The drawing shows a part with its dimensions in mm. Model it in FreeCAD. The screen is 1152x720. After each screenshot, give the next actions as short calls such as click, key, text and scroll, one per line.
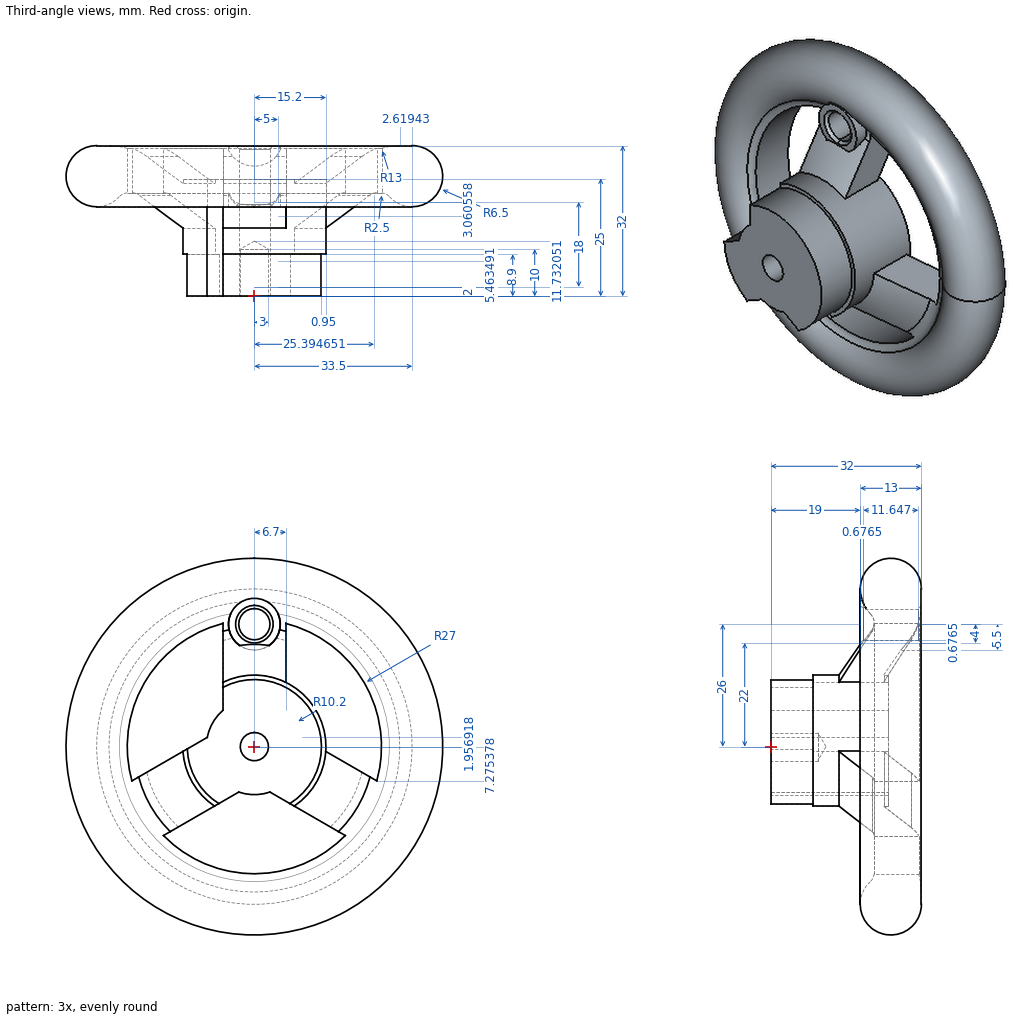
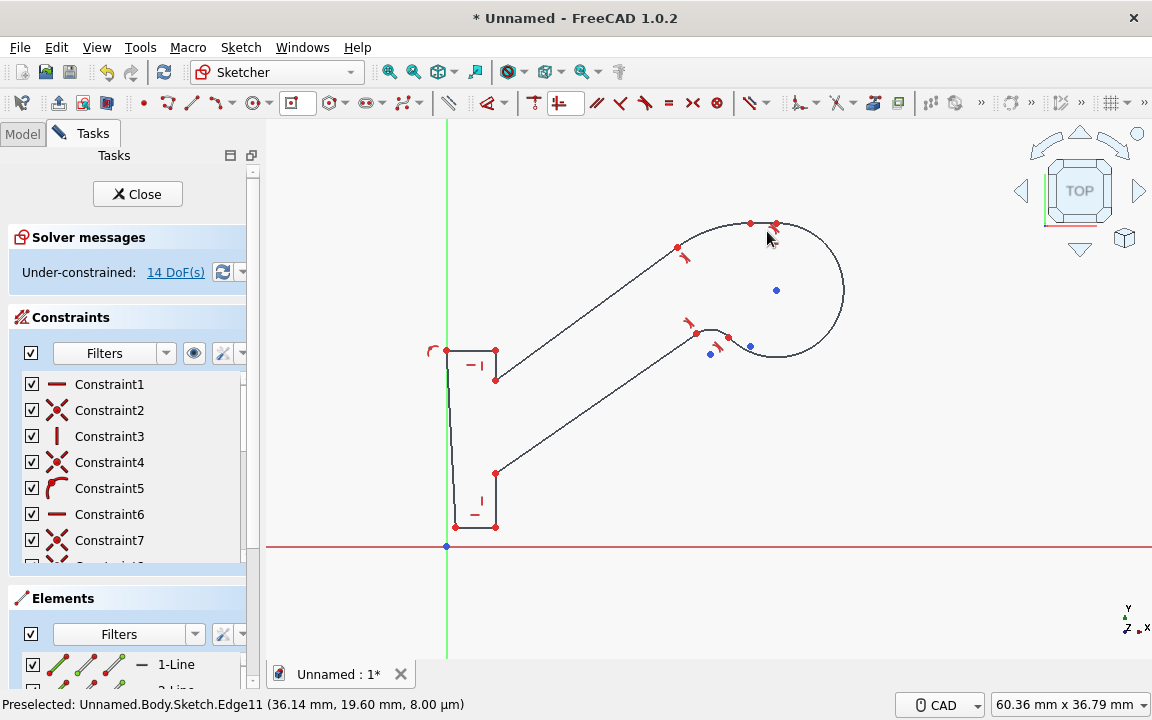
scroll(453, 475, up, 4)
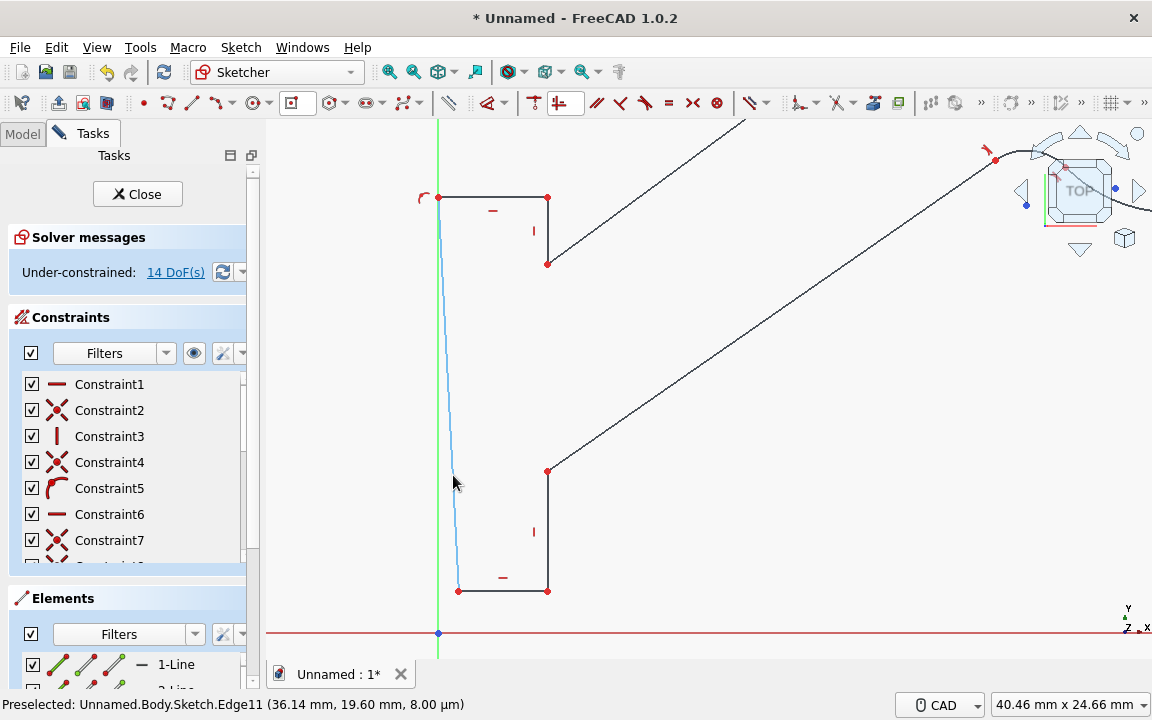
click(453, 473)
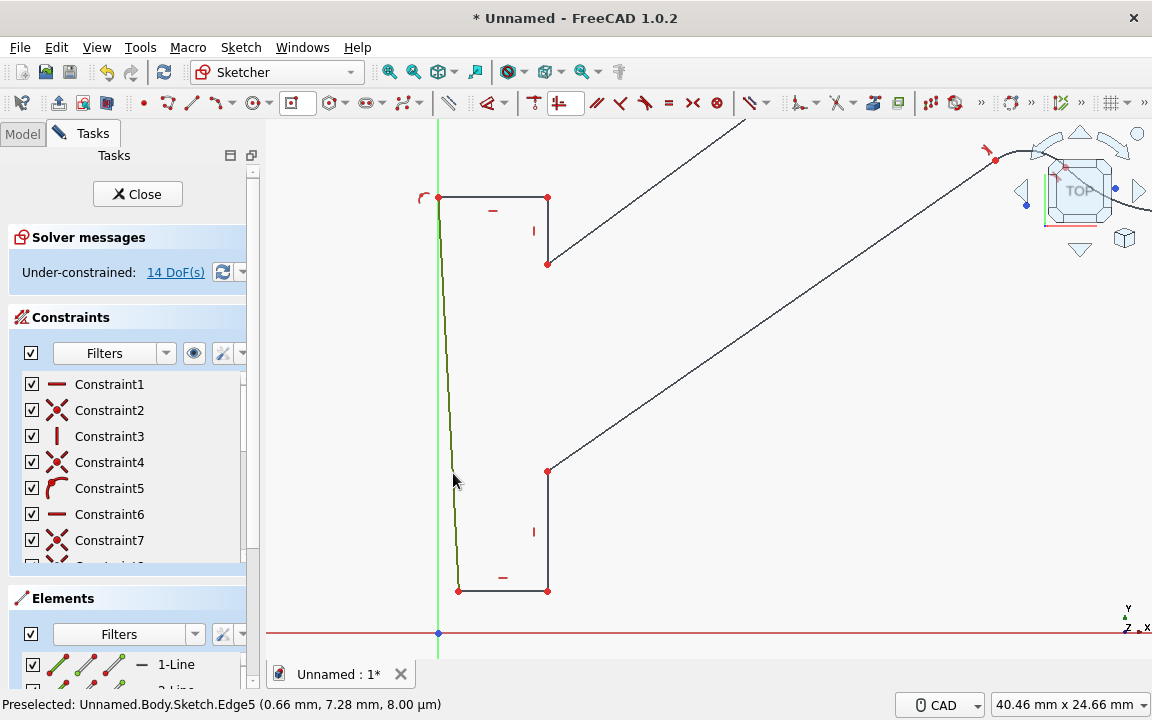
click(578, 104)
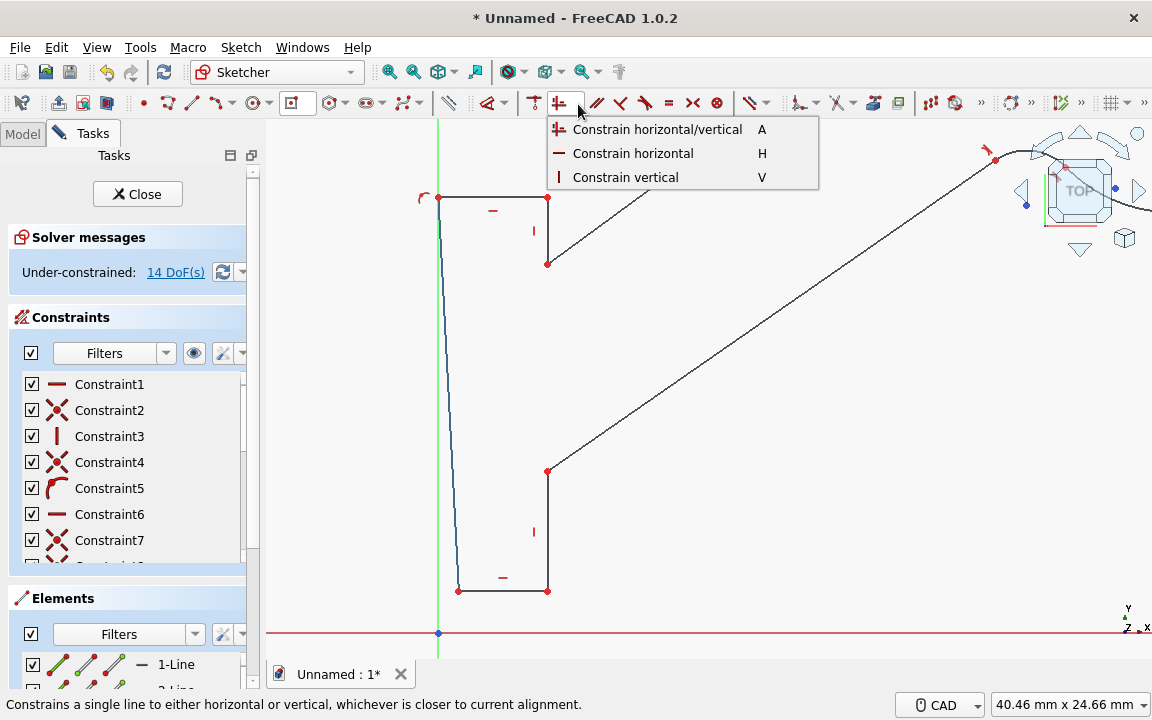
click(683, 177)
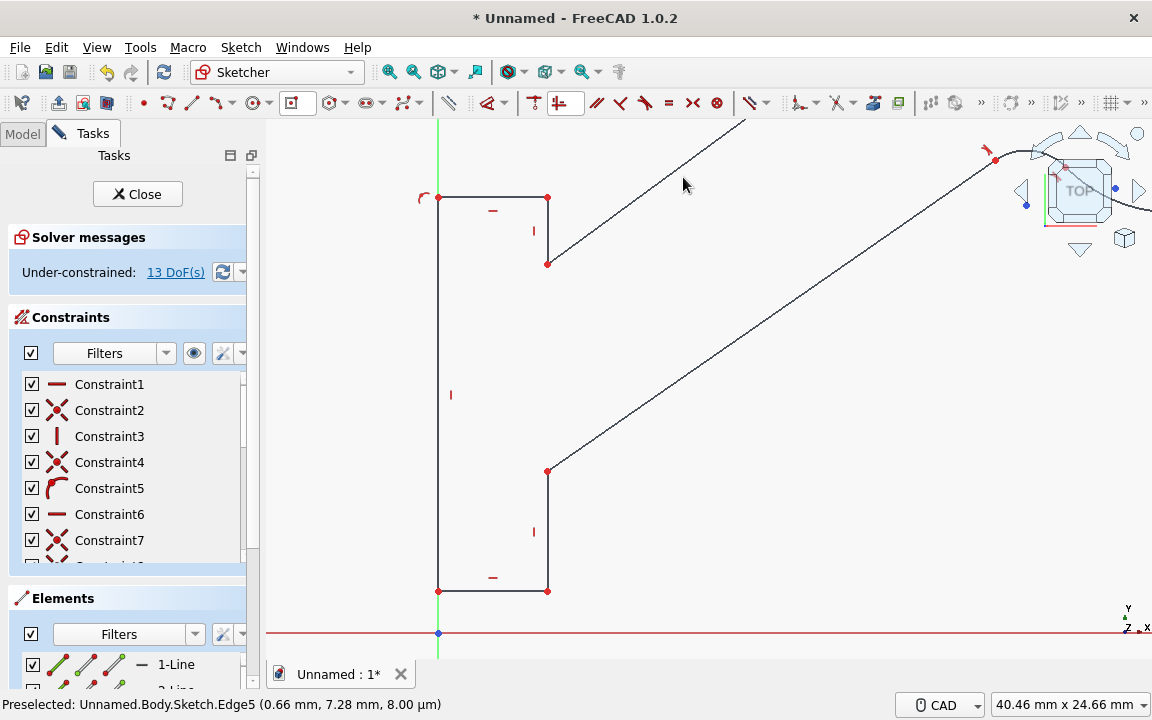
click(488, 104)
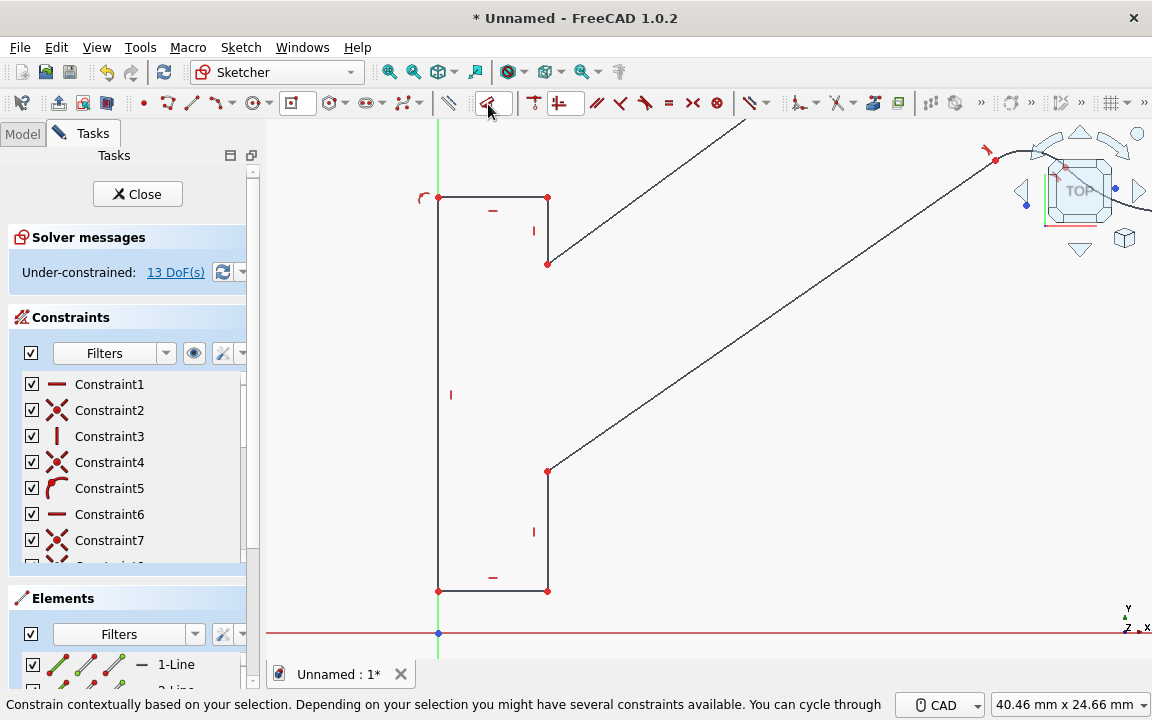
scroll(453, 475, down, 4)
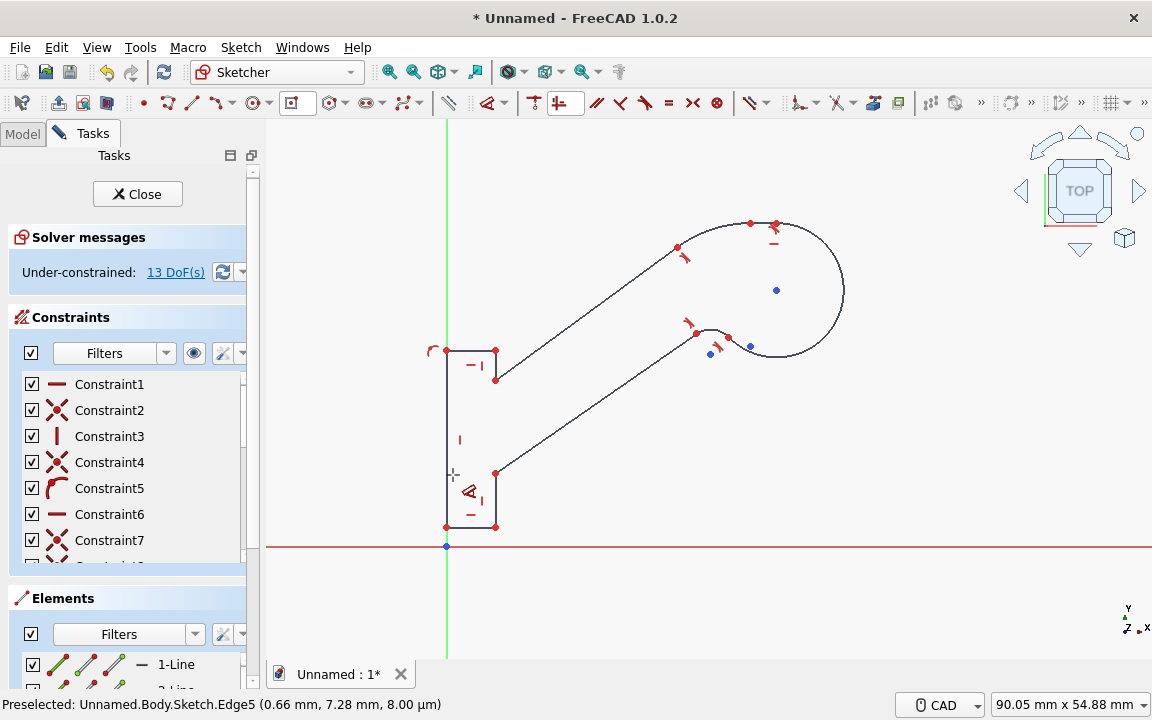
click(727, 225)
click(721, 194)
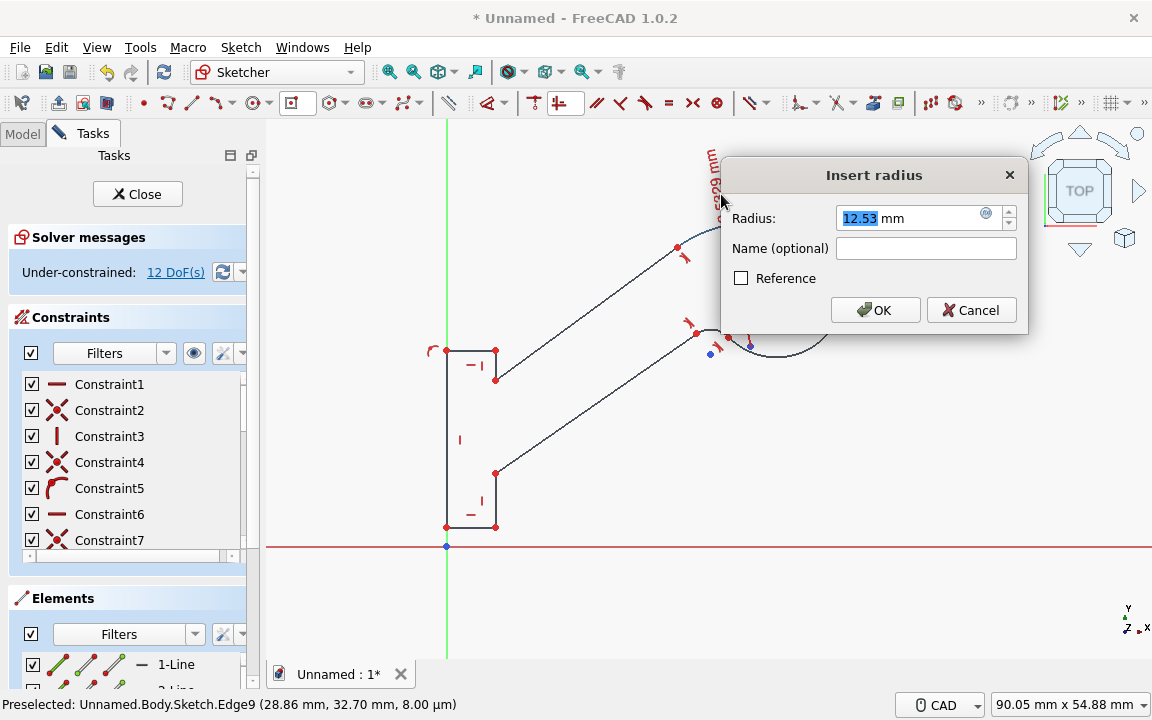
text(13)
key(Return)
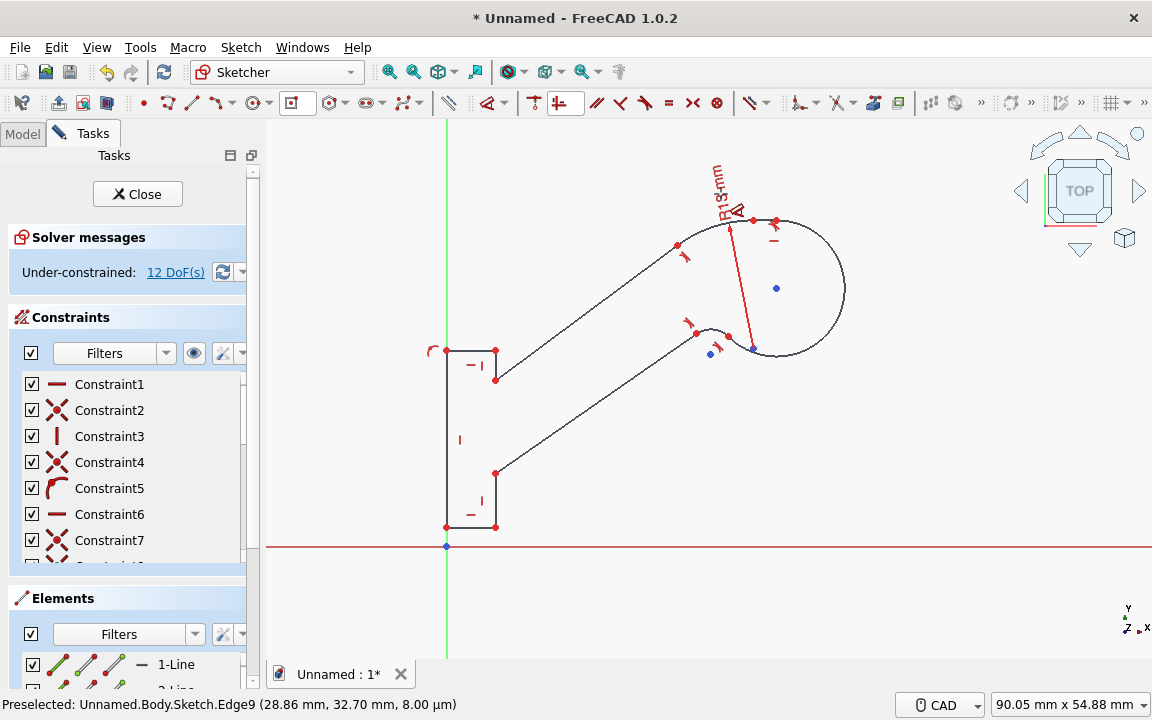
scroll(720, 331, up, 3)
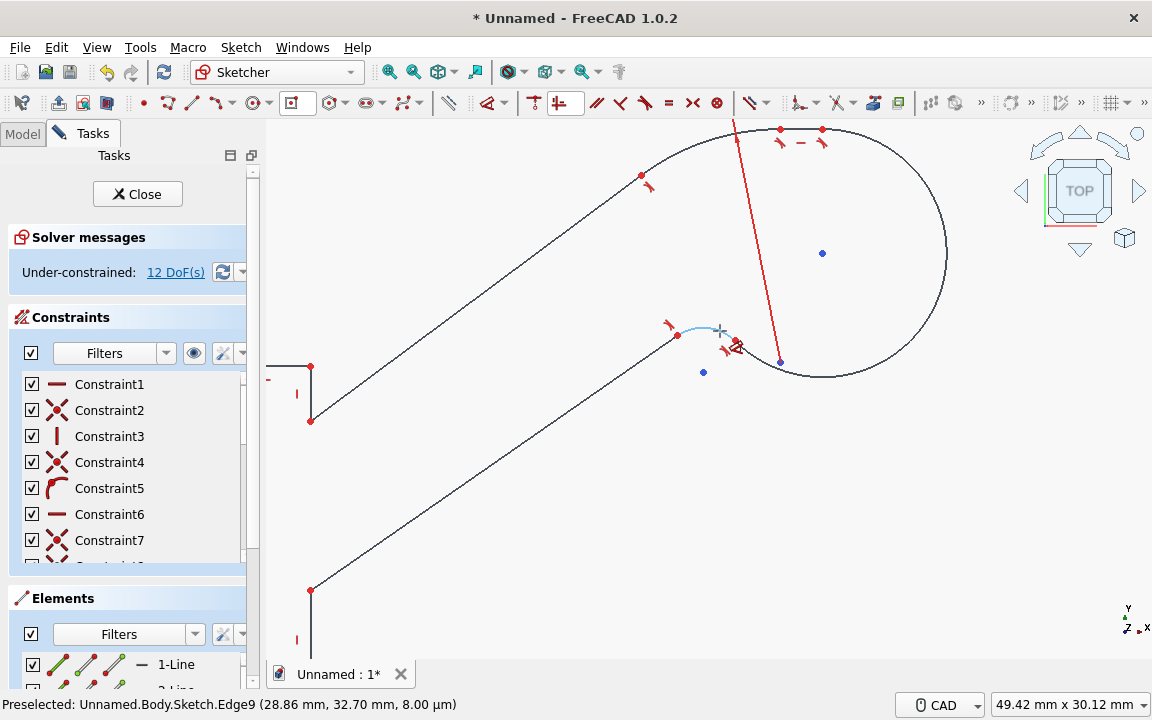
click(719, 331)
click(730, 301)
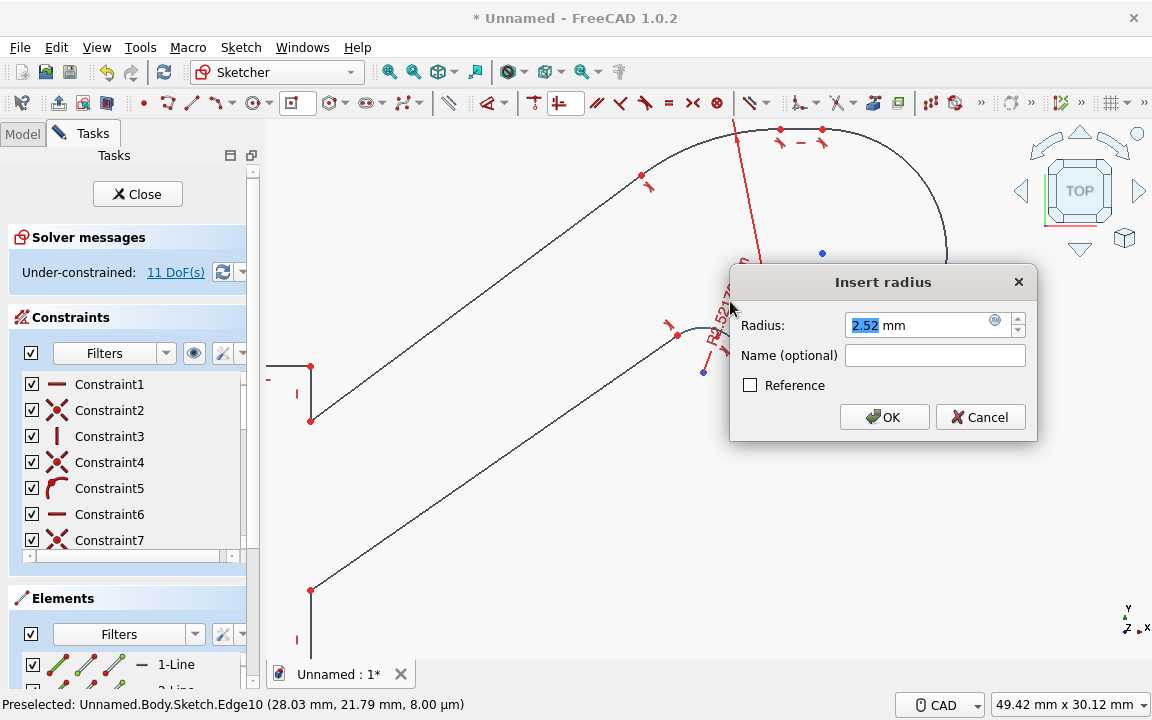
text(2.5)
key(Return)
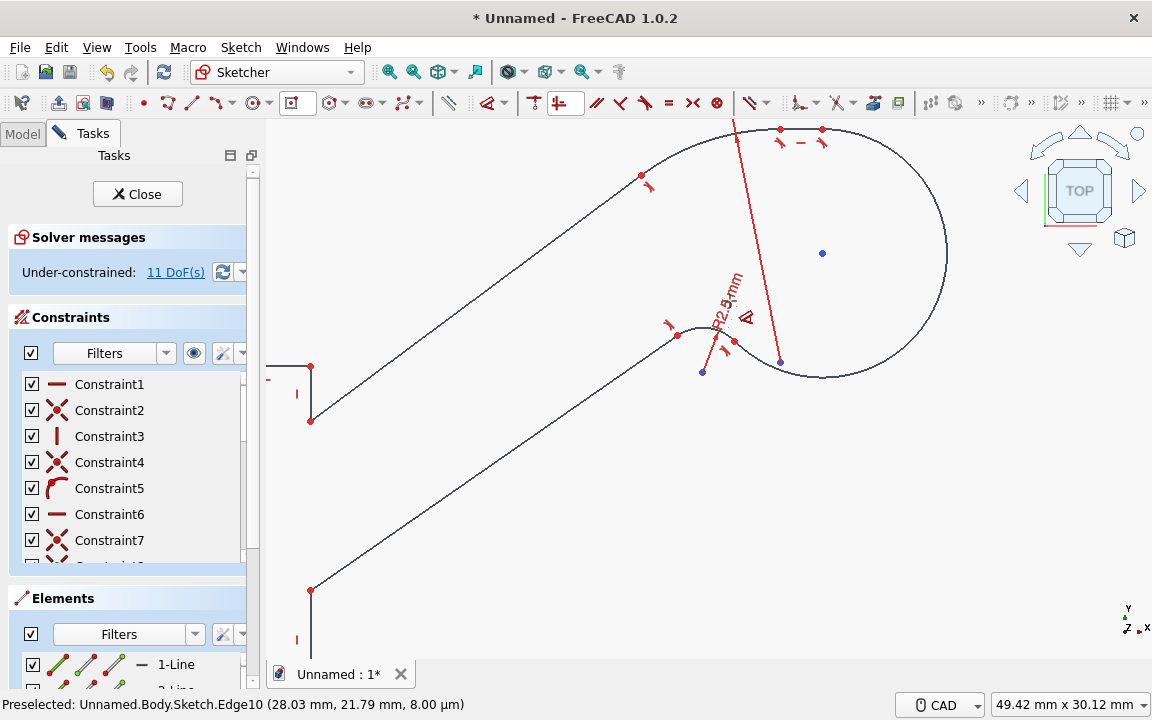
click(870, 368)
click(882, 398)